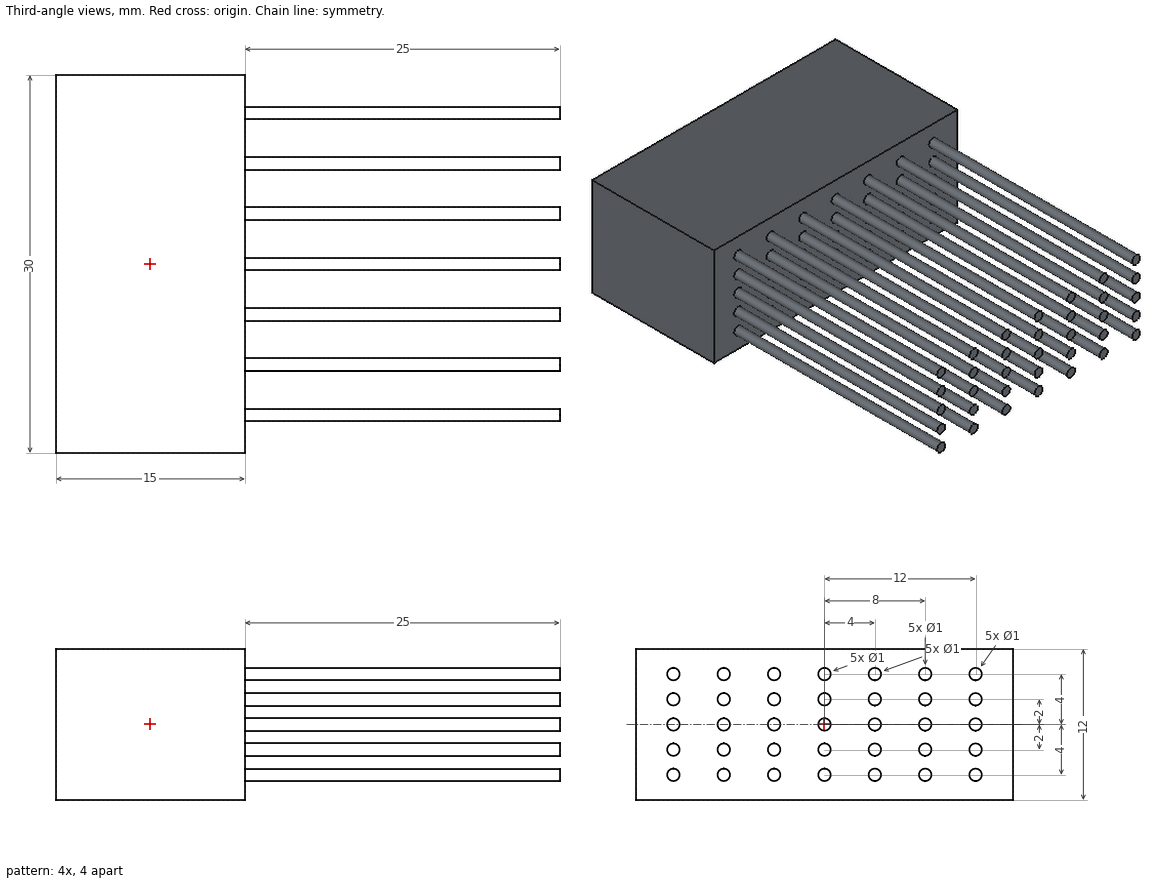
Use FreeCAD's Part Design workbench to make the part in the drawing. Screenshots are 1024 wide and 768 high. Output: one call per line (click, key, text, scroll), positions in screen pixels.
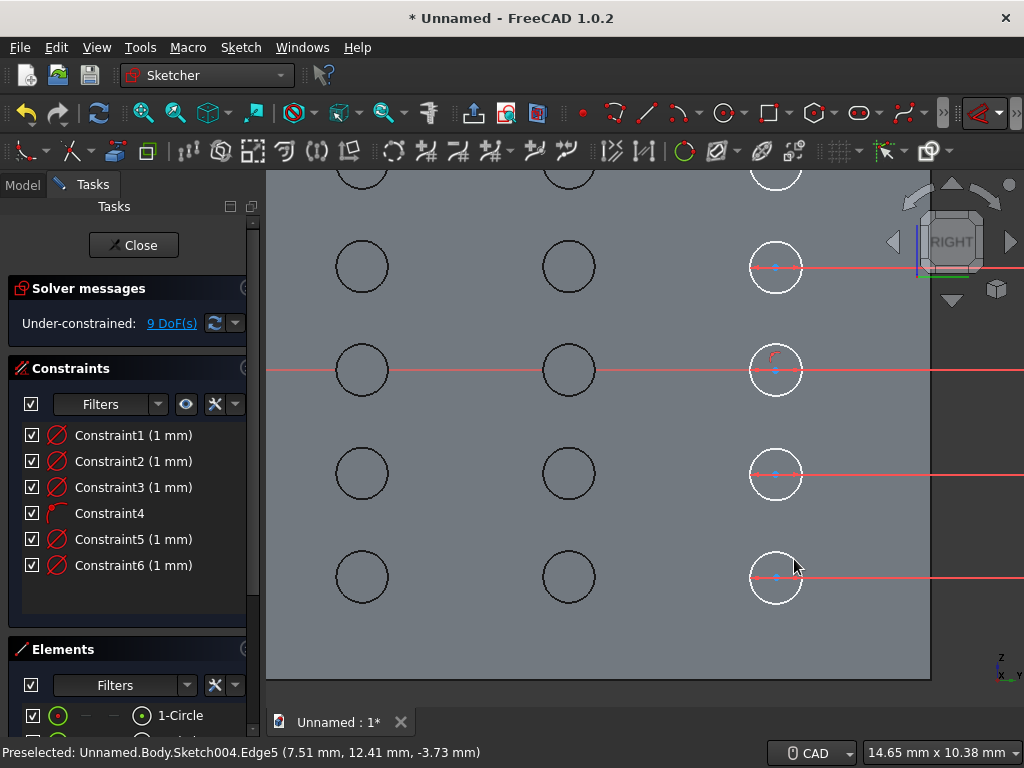
click(776, 268)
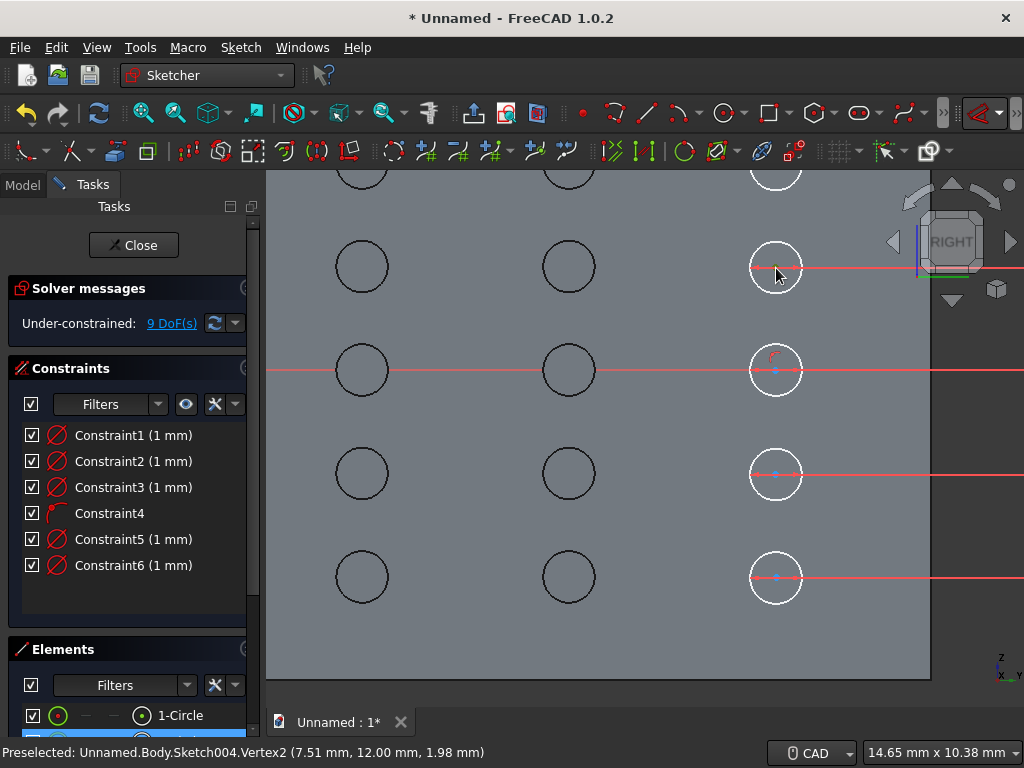
click(776, 475)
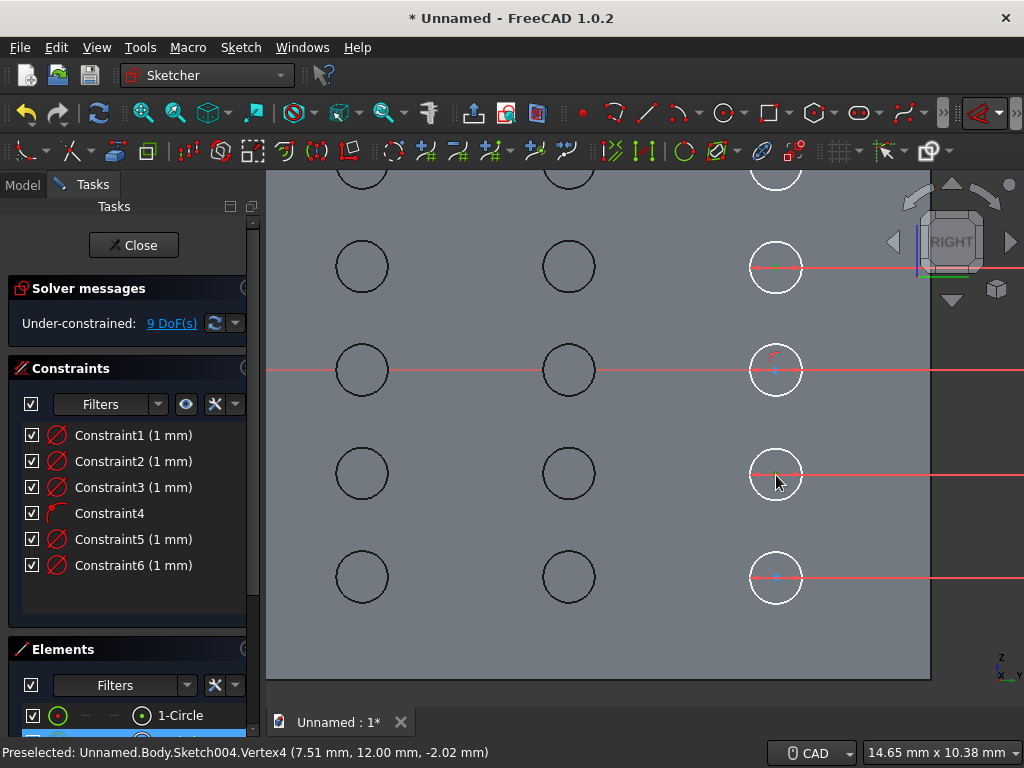
click(334, 370)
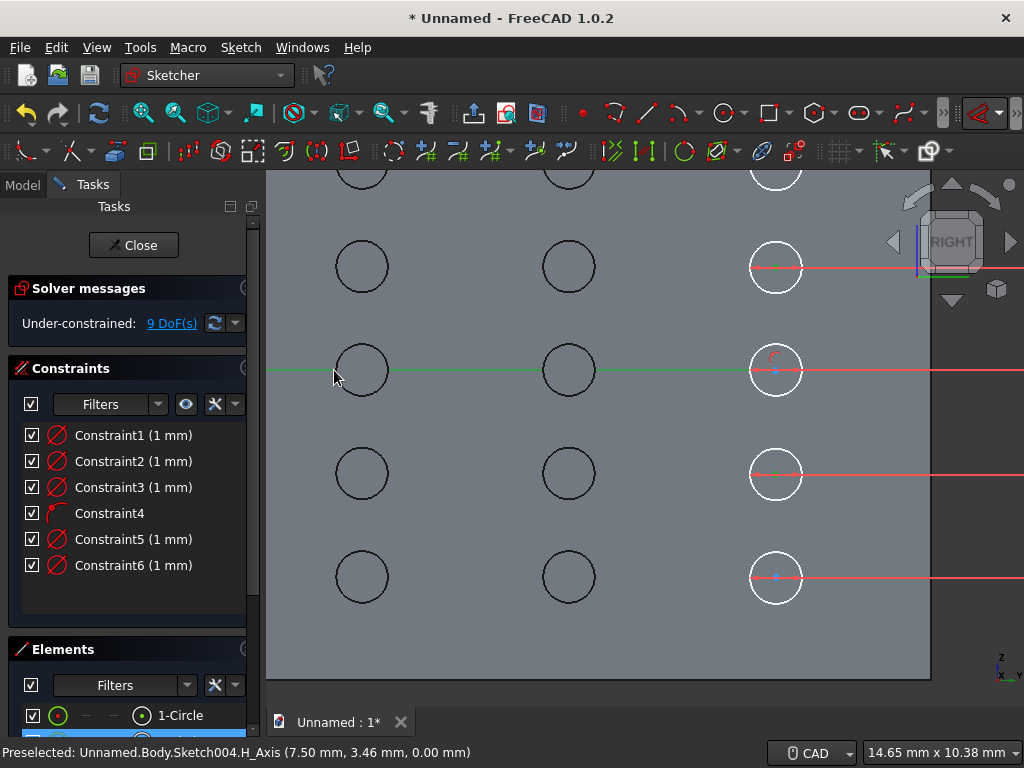
key(s)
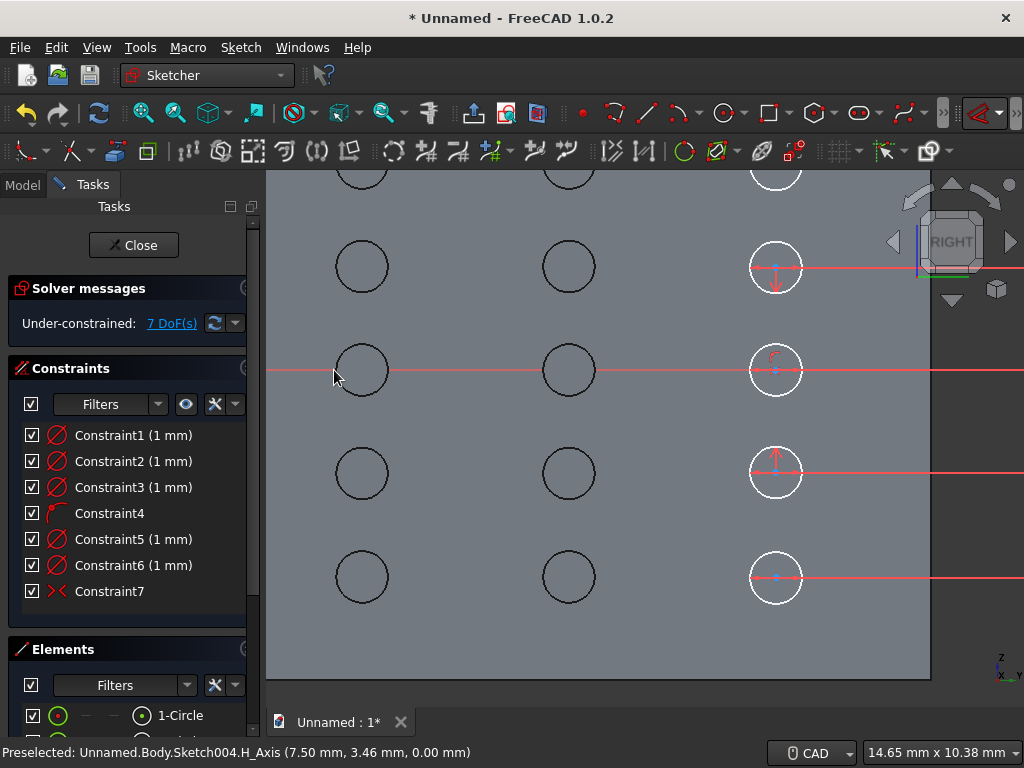
scroll(776, 578, down, 2)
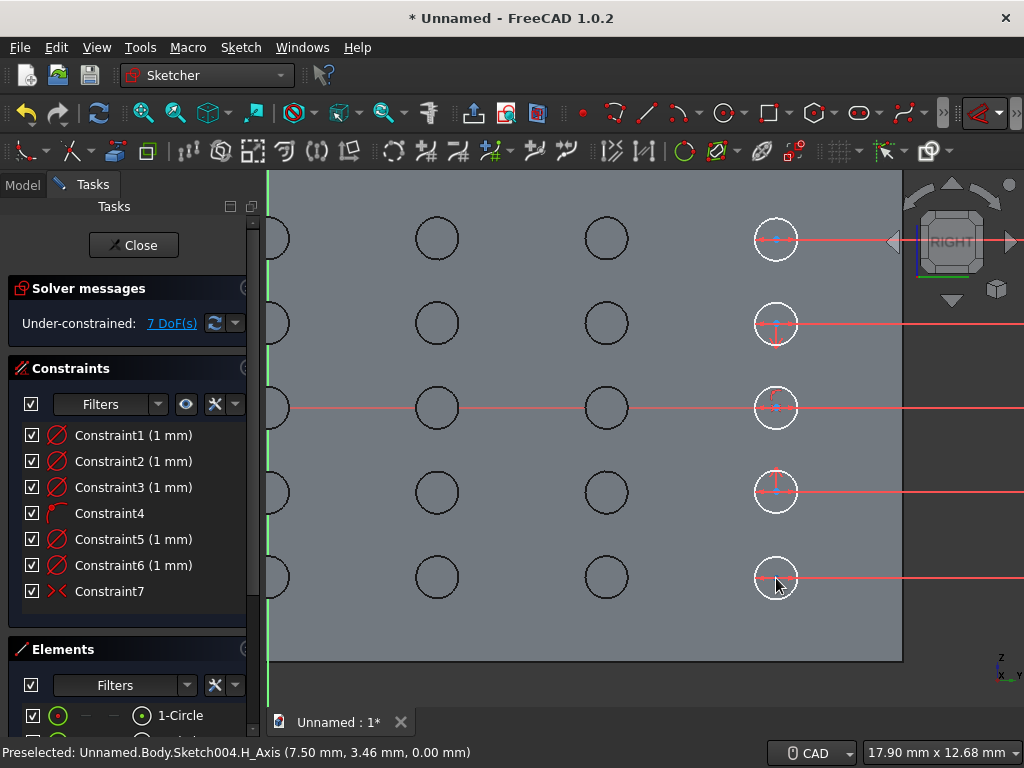
click(776, 301)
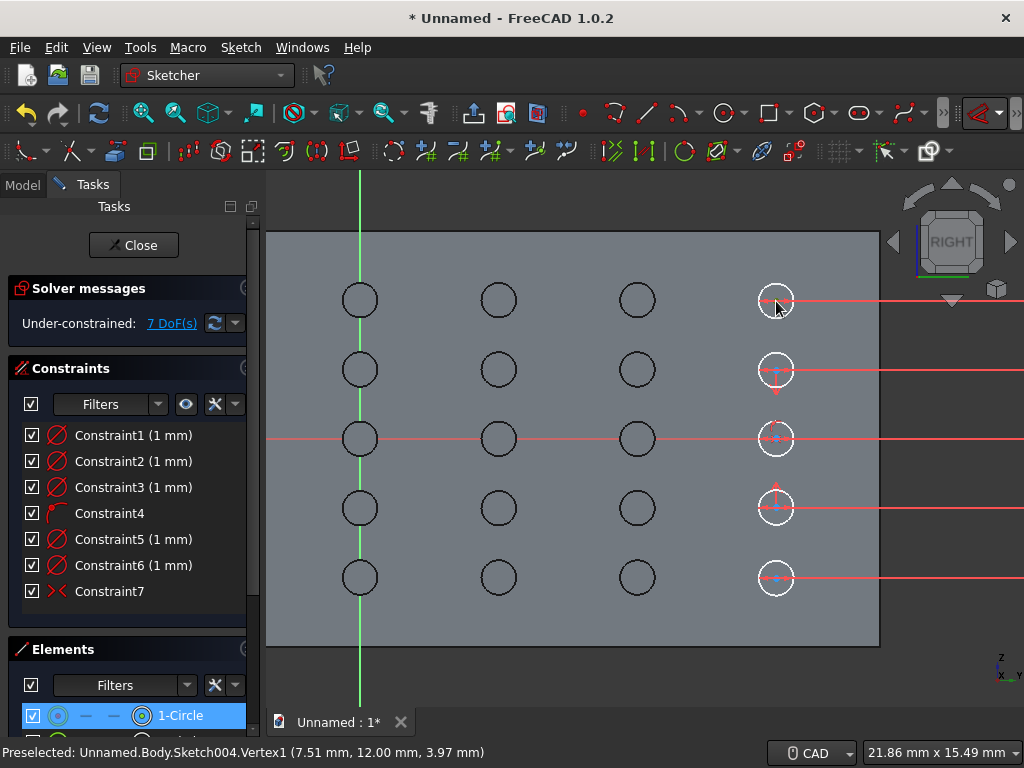
click(776, 578)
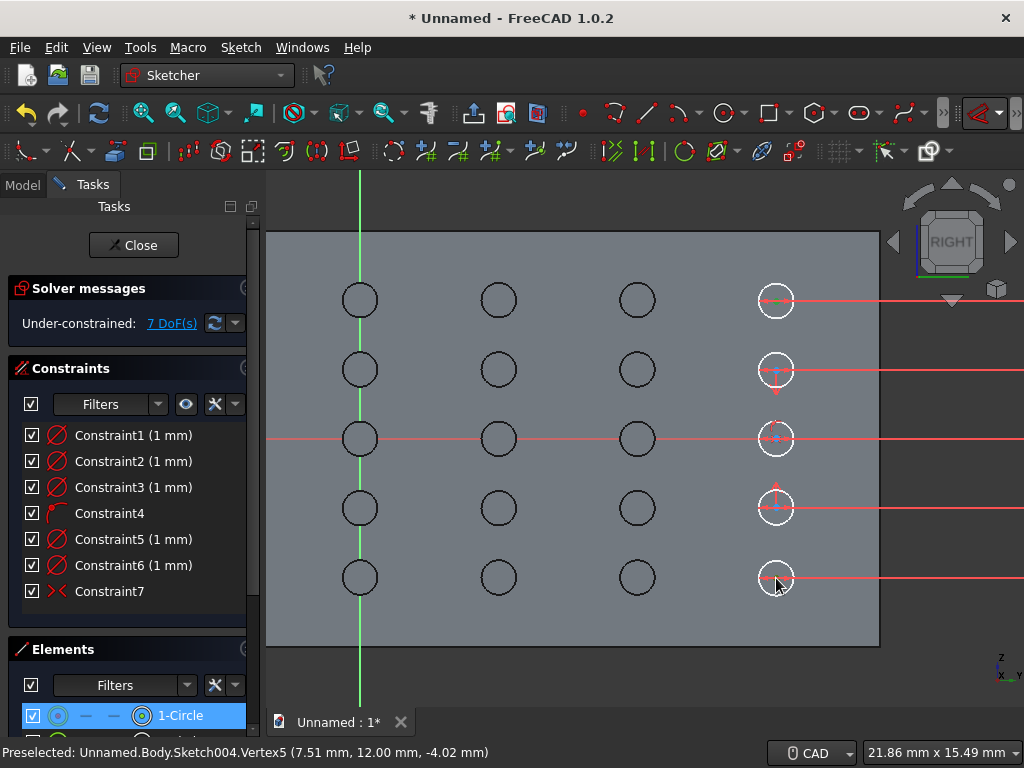
click(415, 439)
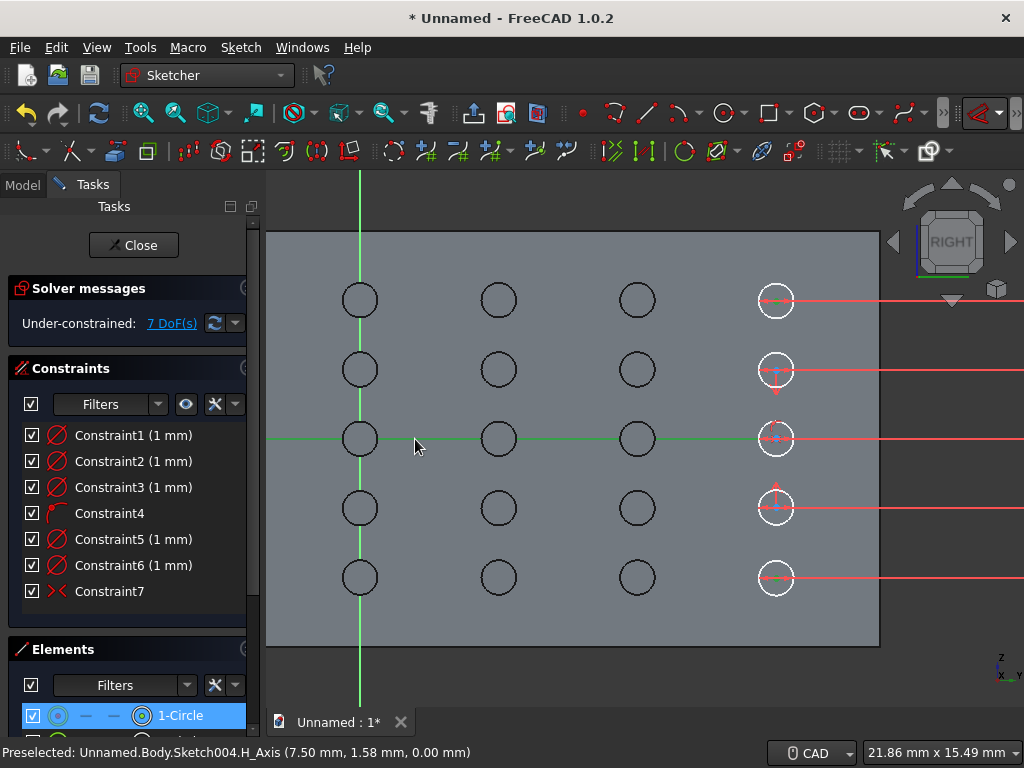
key(s)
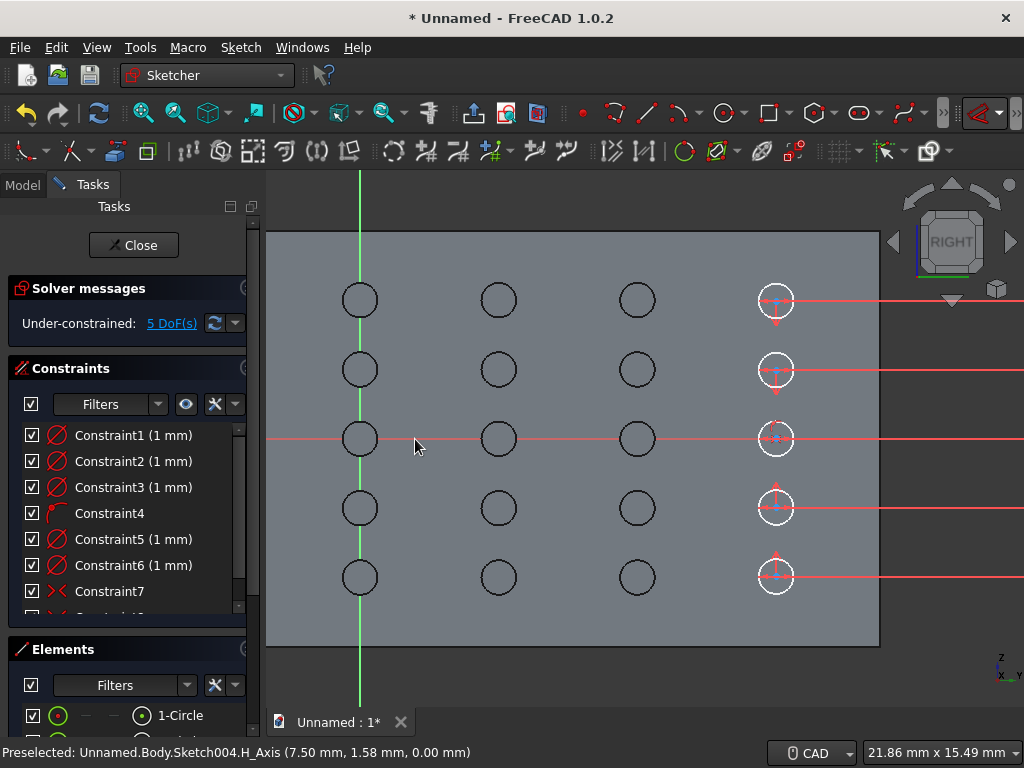
click(776, 301)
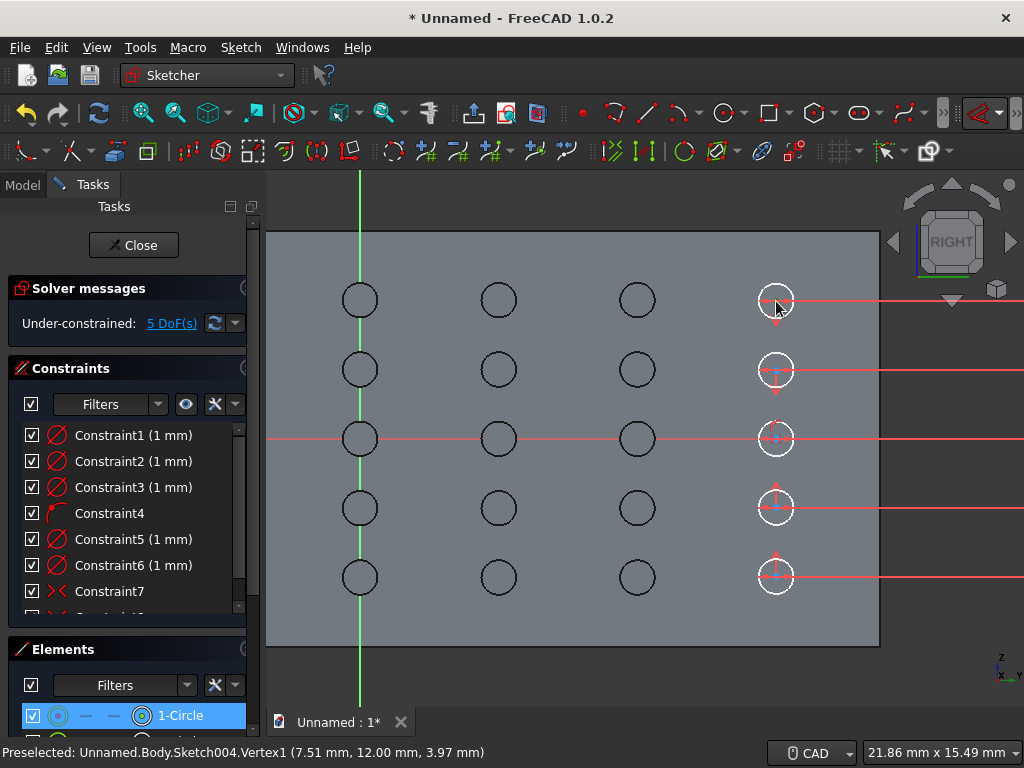
key(i)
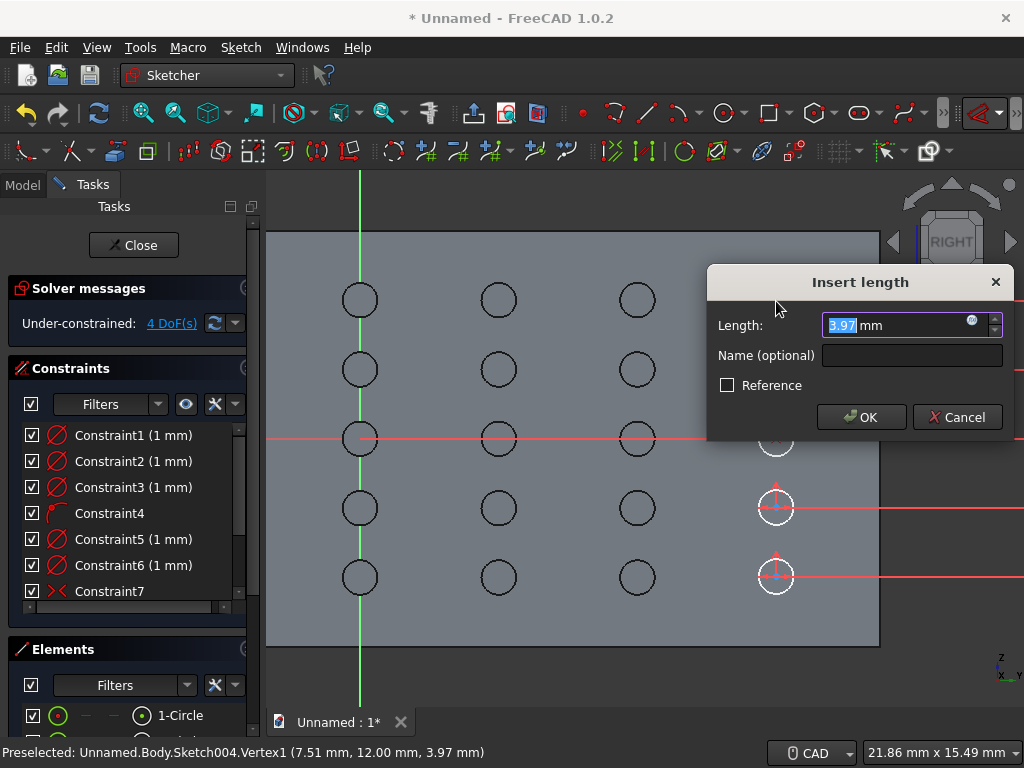
text(4)
key(Return)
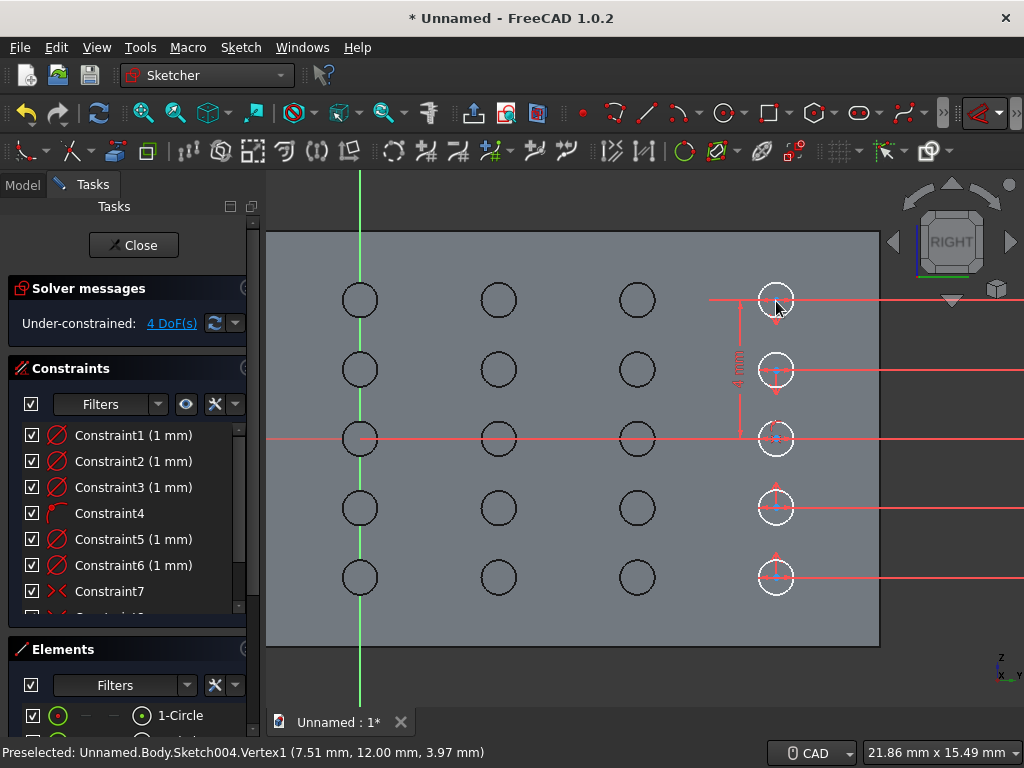
click(776, 370)